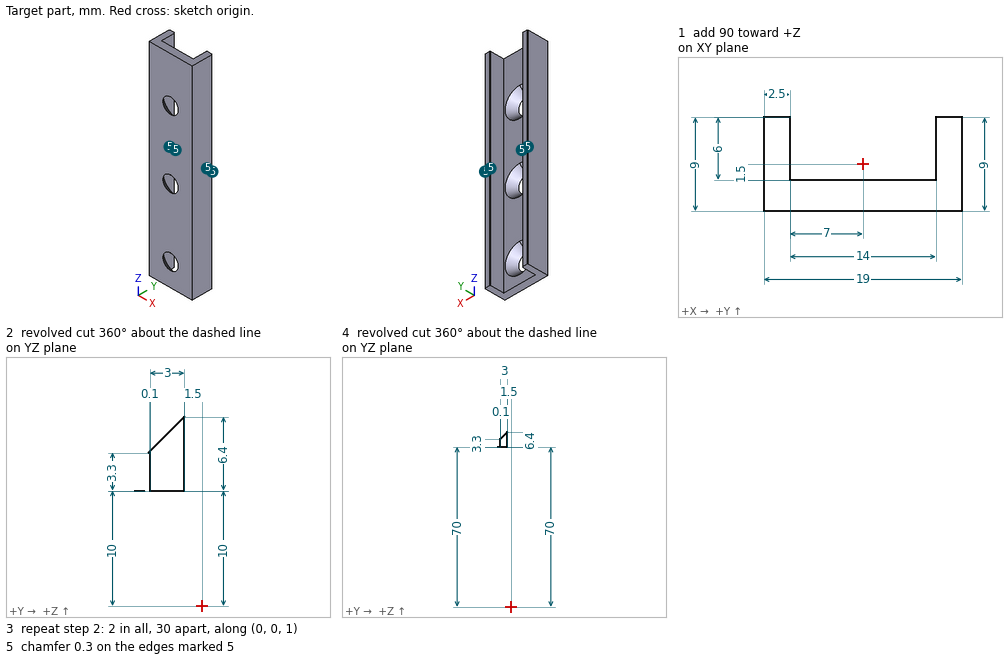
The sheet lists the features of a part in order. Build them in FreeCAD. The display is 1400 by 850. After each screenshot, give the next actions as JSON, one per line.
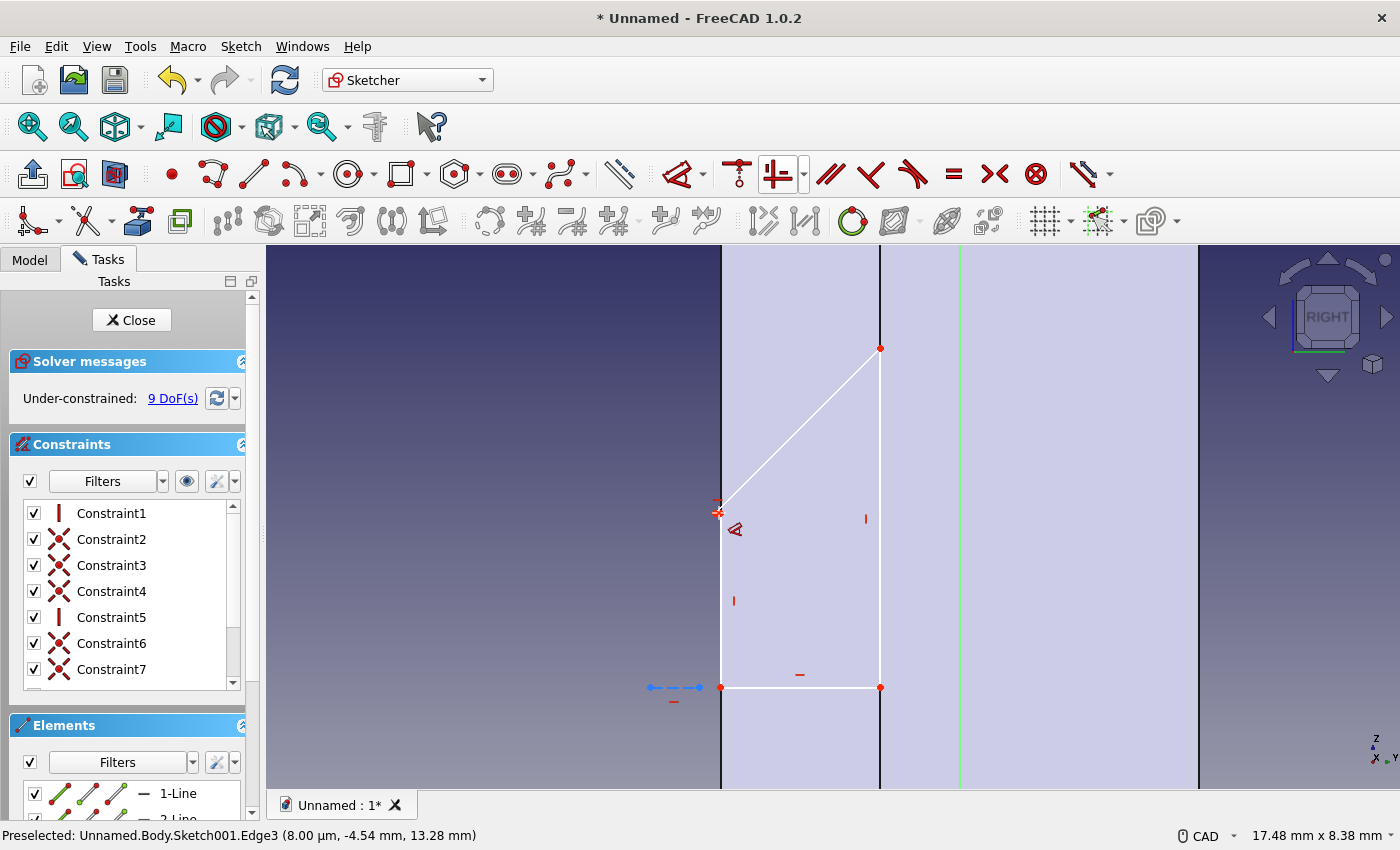
{"action": "left_click", "coordinate": [769, 688]}
{"action": "left_click", "coordinate": [801, 722]}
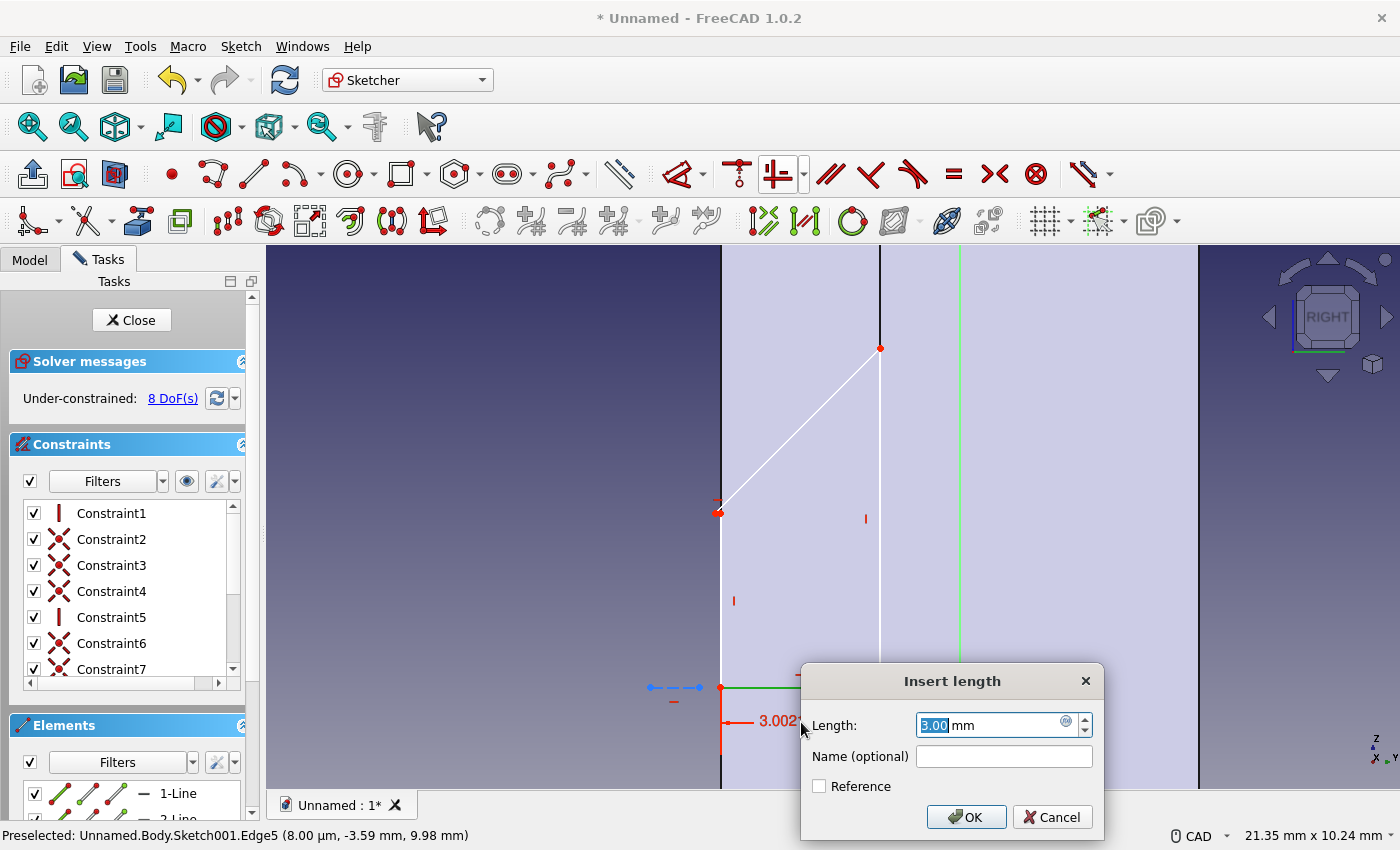
{"action": "type", "text": "3"}
{"action": "key", "text": "Return"}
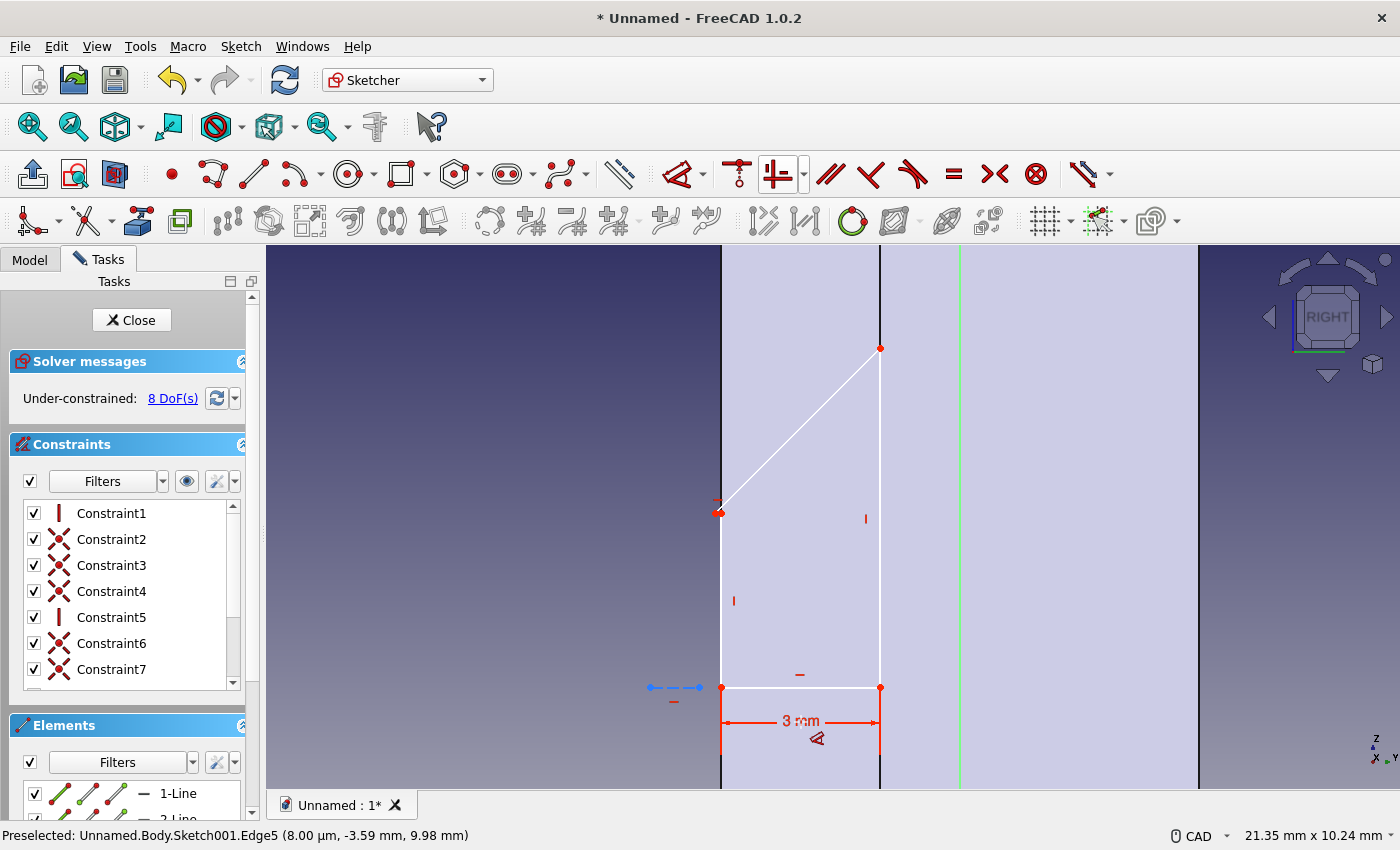
{"action": "left_click", "coordinate": [880, 586]}
{"action": "left_click", "coordinate": [914, 518]}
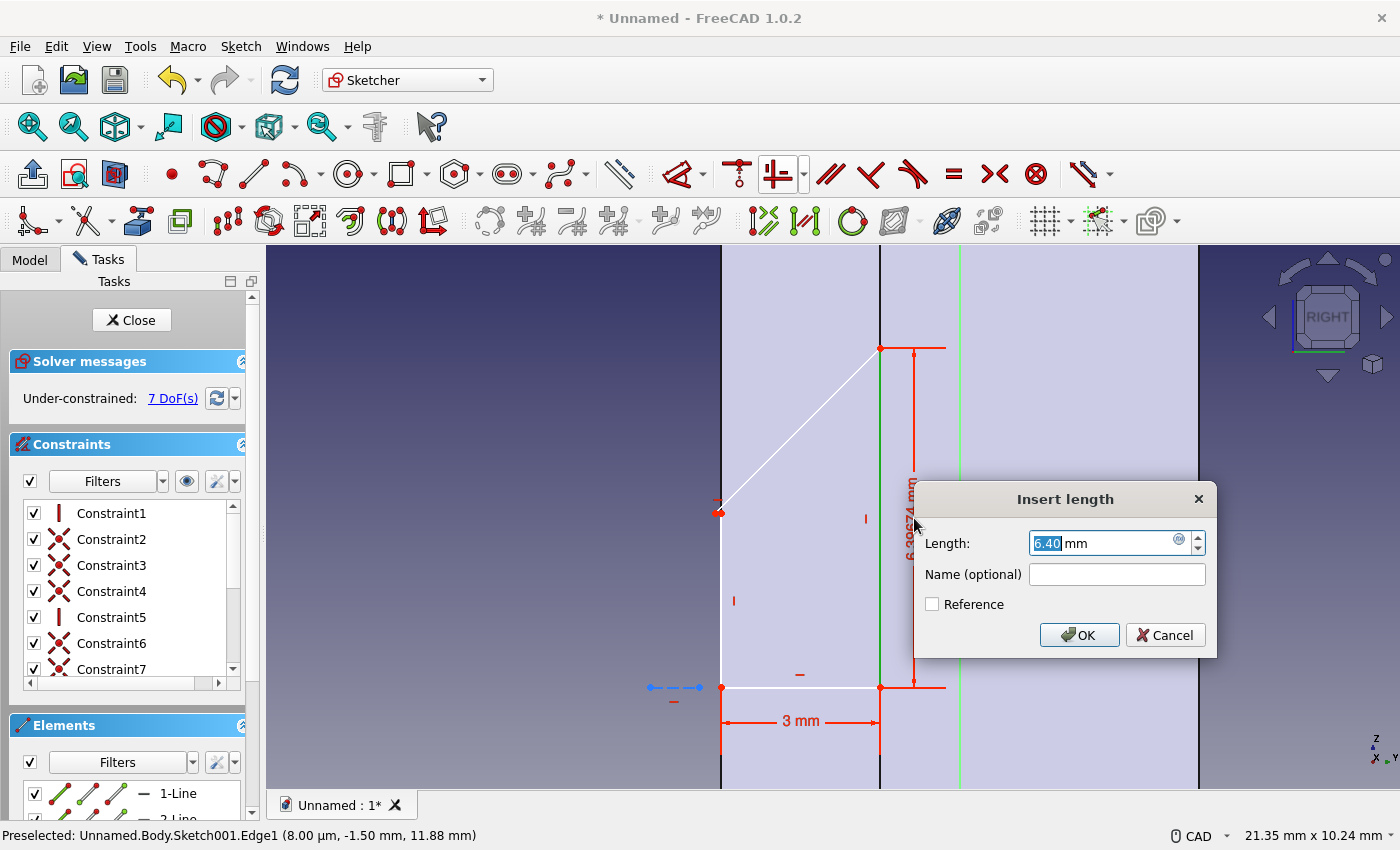
{"action": "type", "text": "6.4"}
{"action": "key", "text": "Return"}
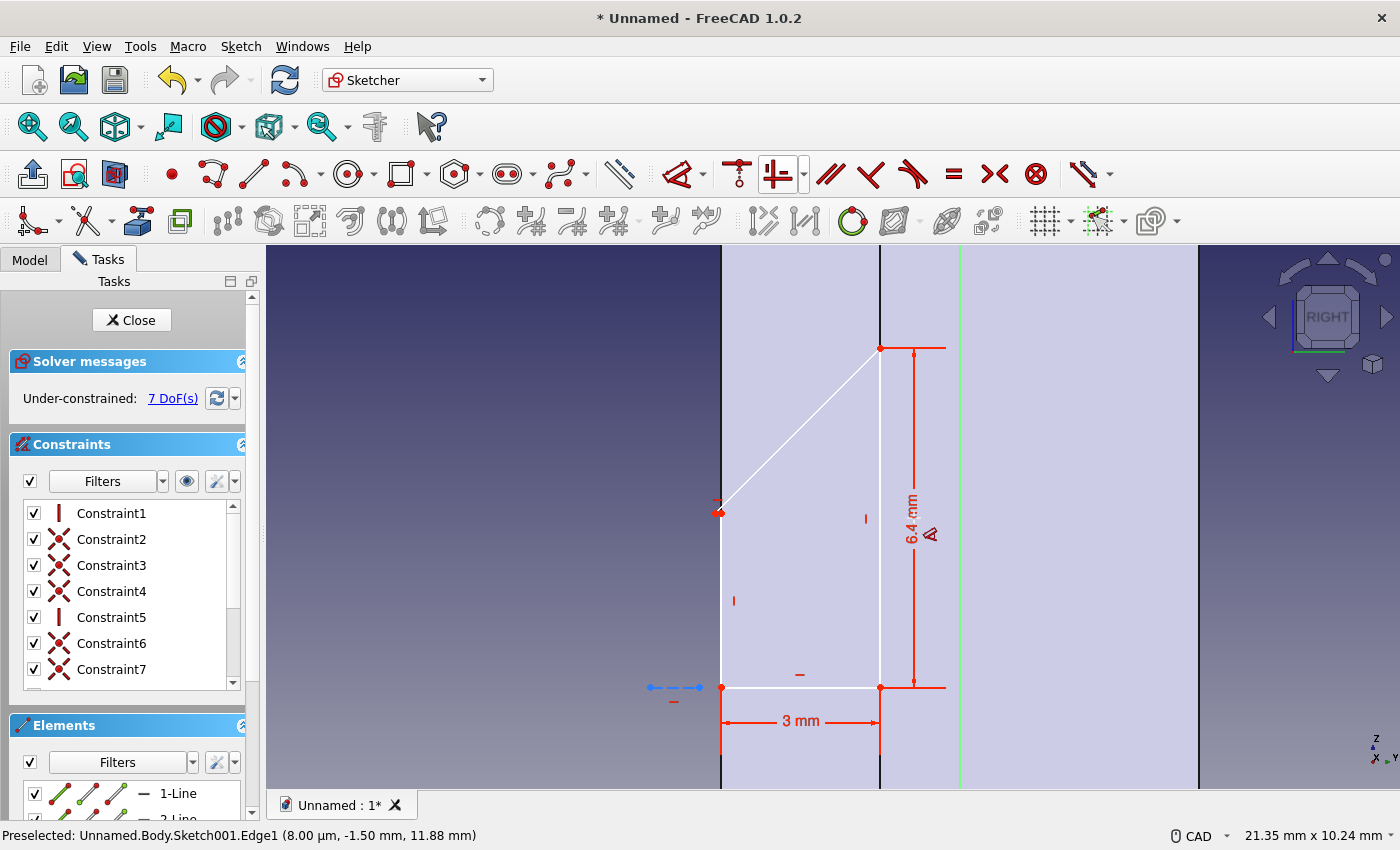
{"action": "scroll", "coordinate": [719, 513], "scroll_direction": "up", "scroll_amount": 11}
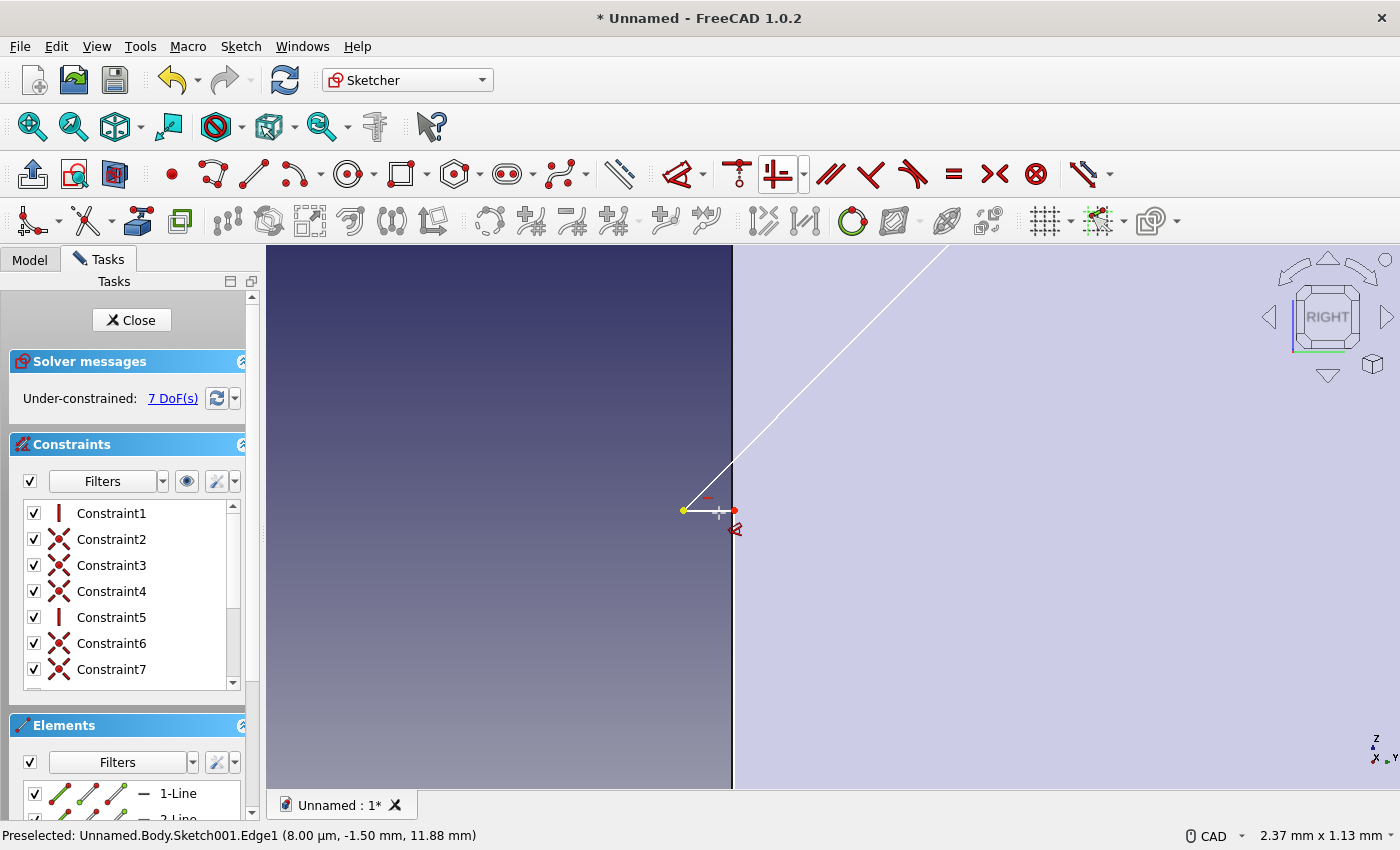
{"action": "left_click", "coordinate": [714, 511]}
{"action": "left_click", "coordinate": [697, 477]}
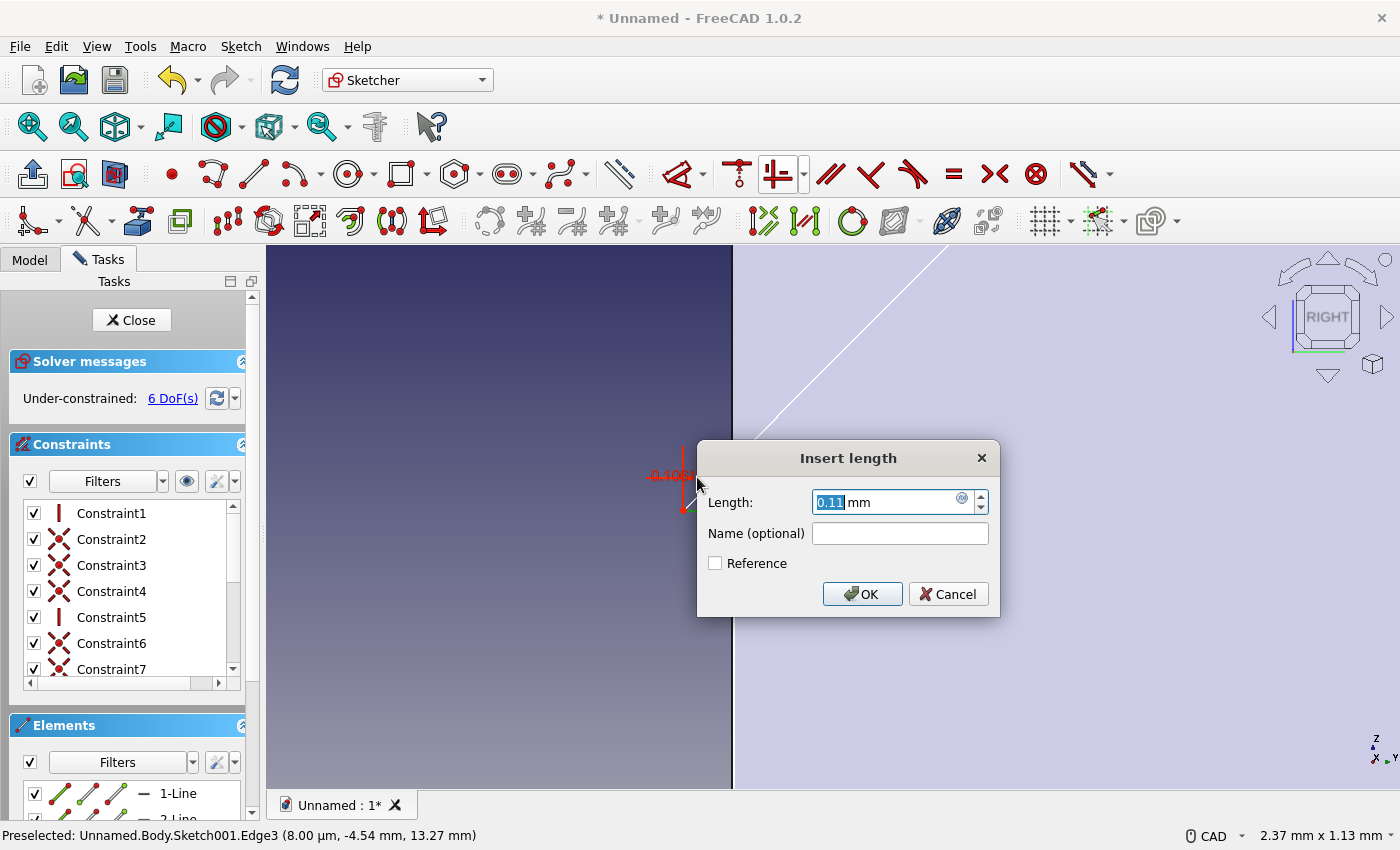
{"action": "type", "text": "0.1"}
{"action": "key", "text": "Return"}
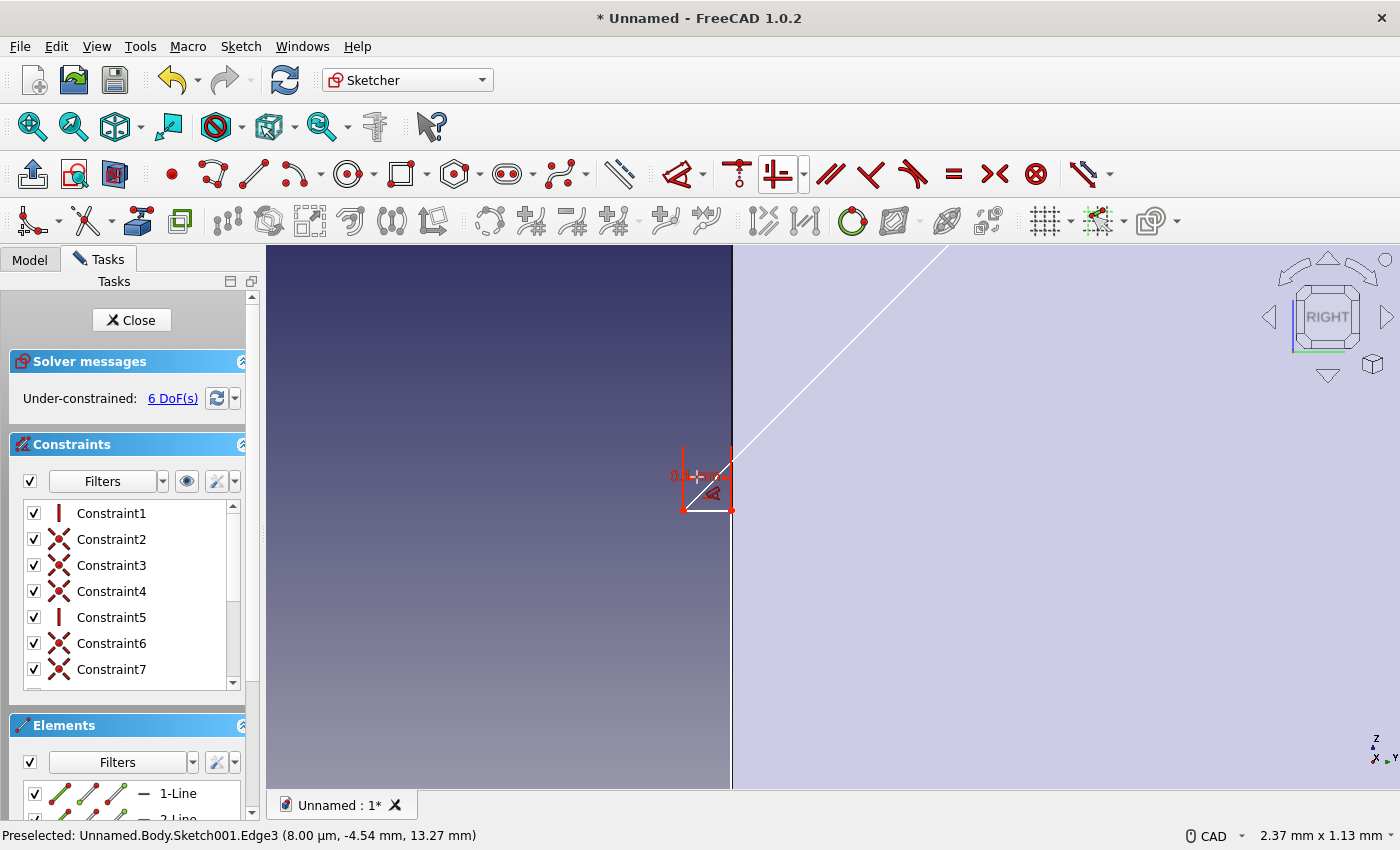
{"action": "scroll", "coordinate": [719, 513], "scroll_direction": "down", "scroll_amount": 11}